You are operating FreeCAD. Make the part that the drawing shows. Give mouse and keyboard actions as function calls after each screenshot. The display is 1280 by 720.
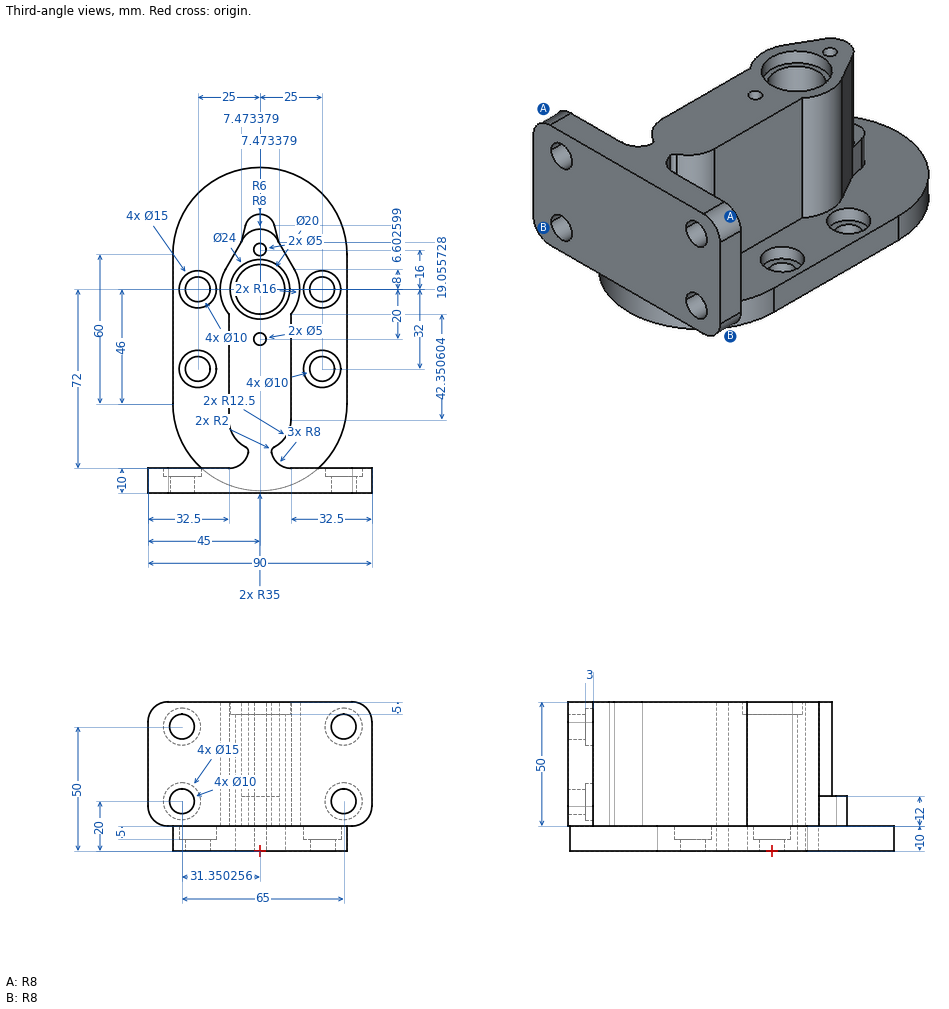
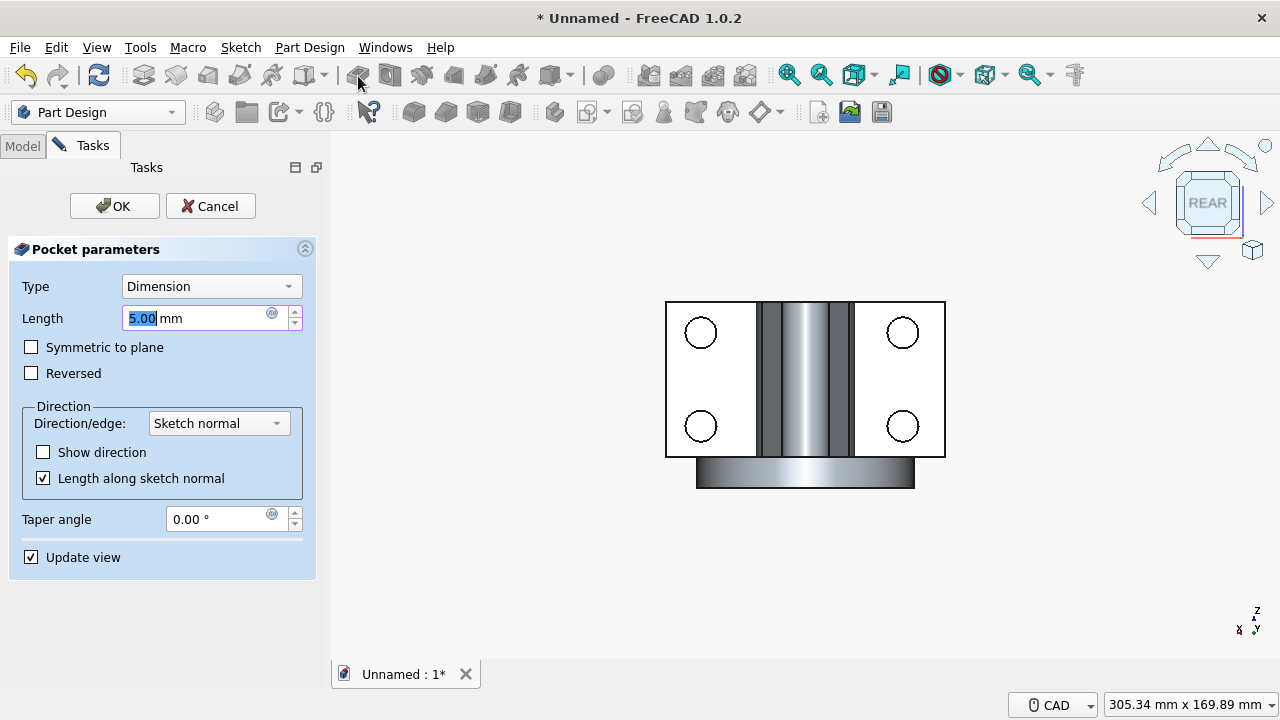
text(20)
key(Tab)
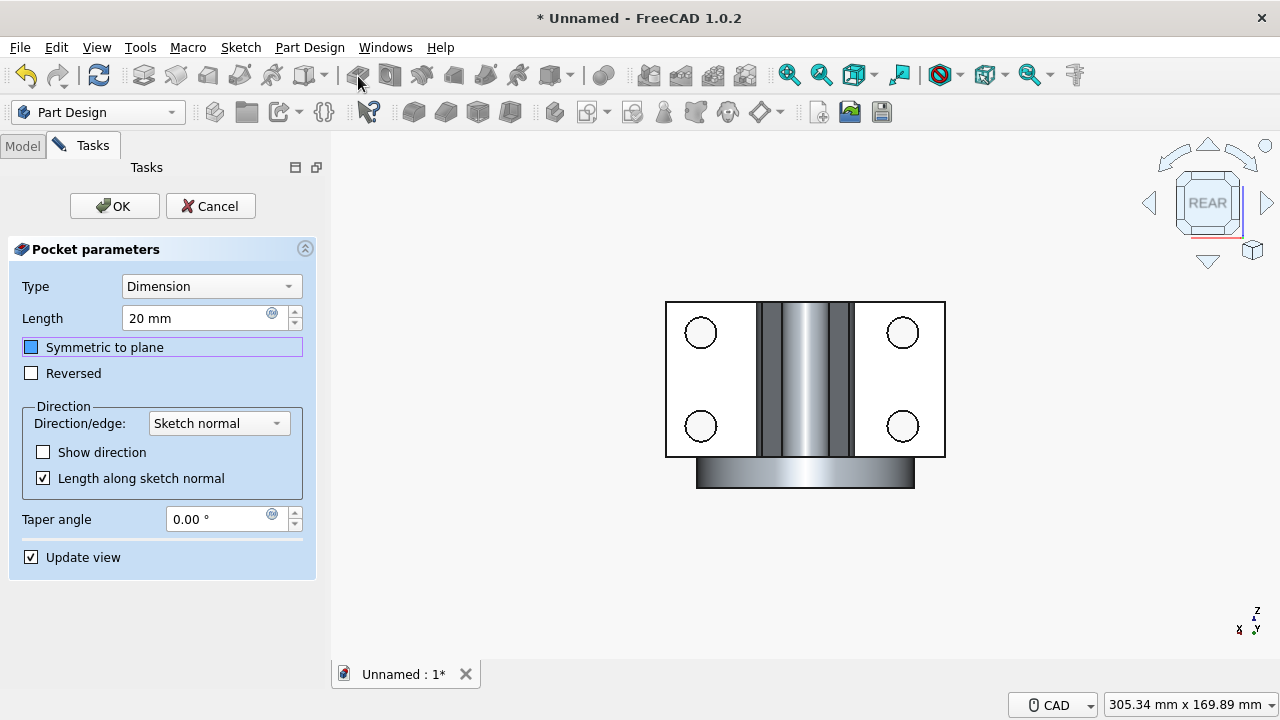
click(115, 206)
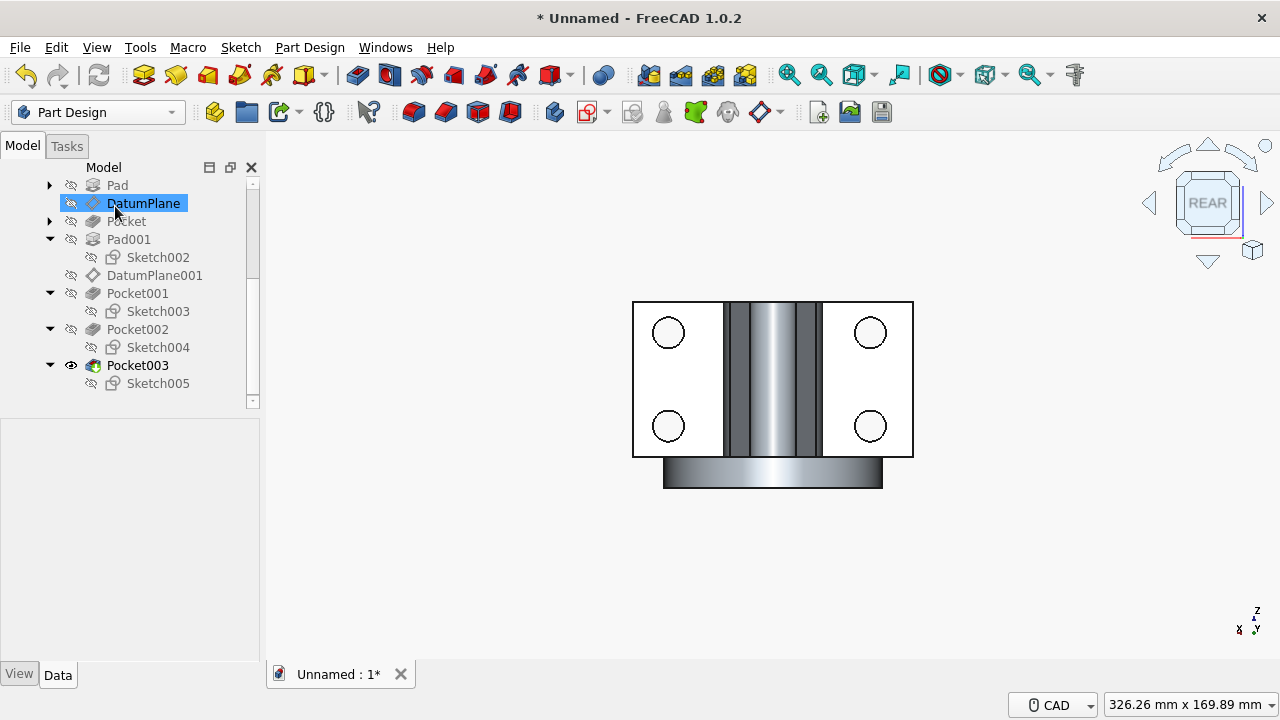
click(790, 76)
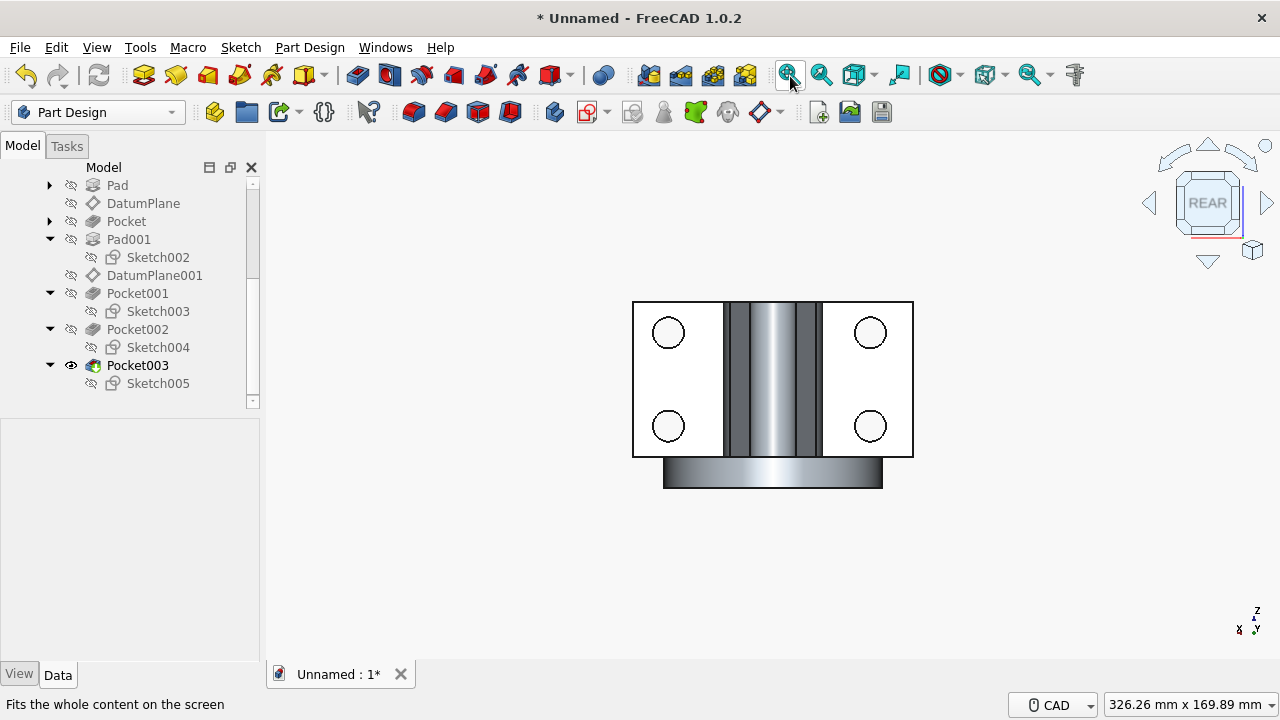
click(848, 378)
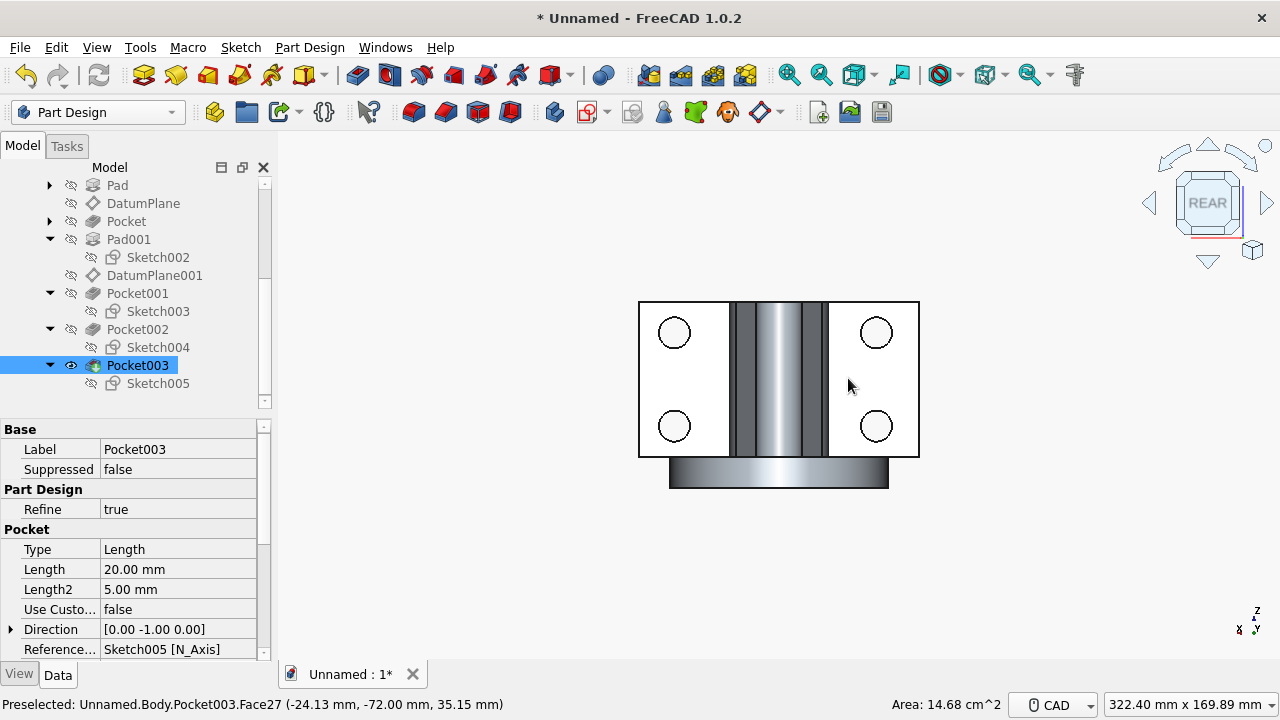
click(588, 112)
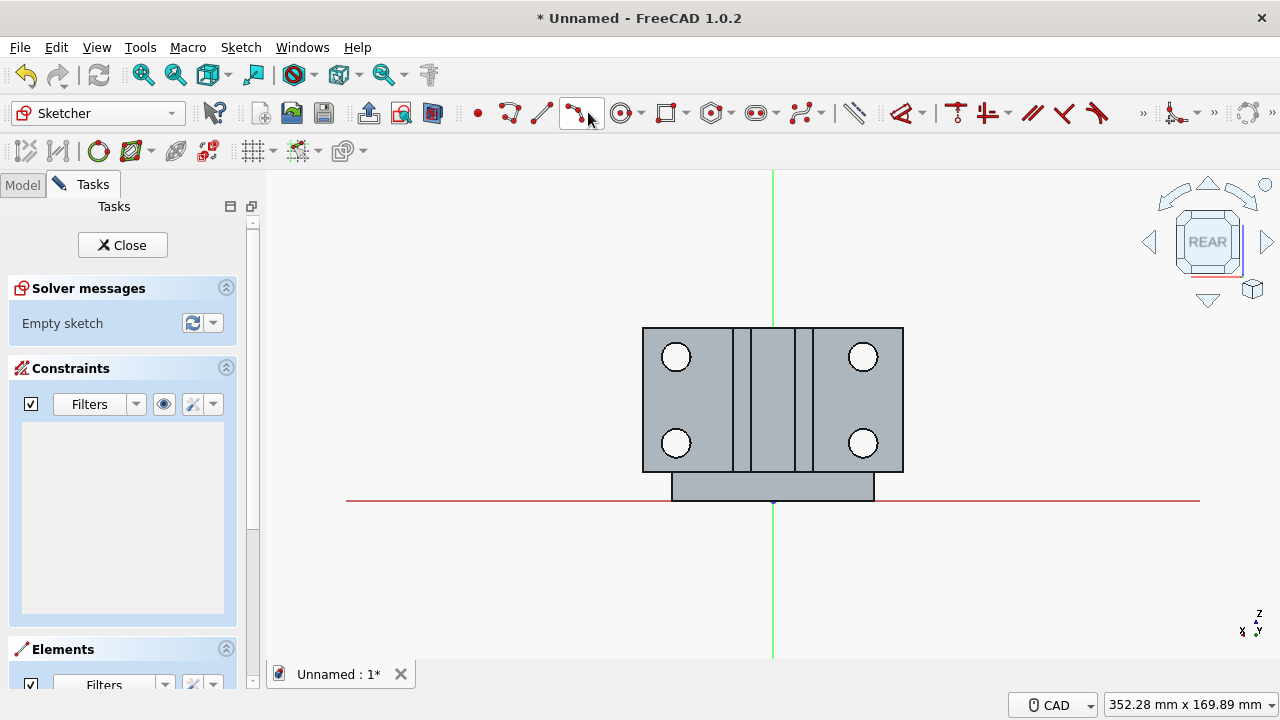
scroll(849, 422, up, 3)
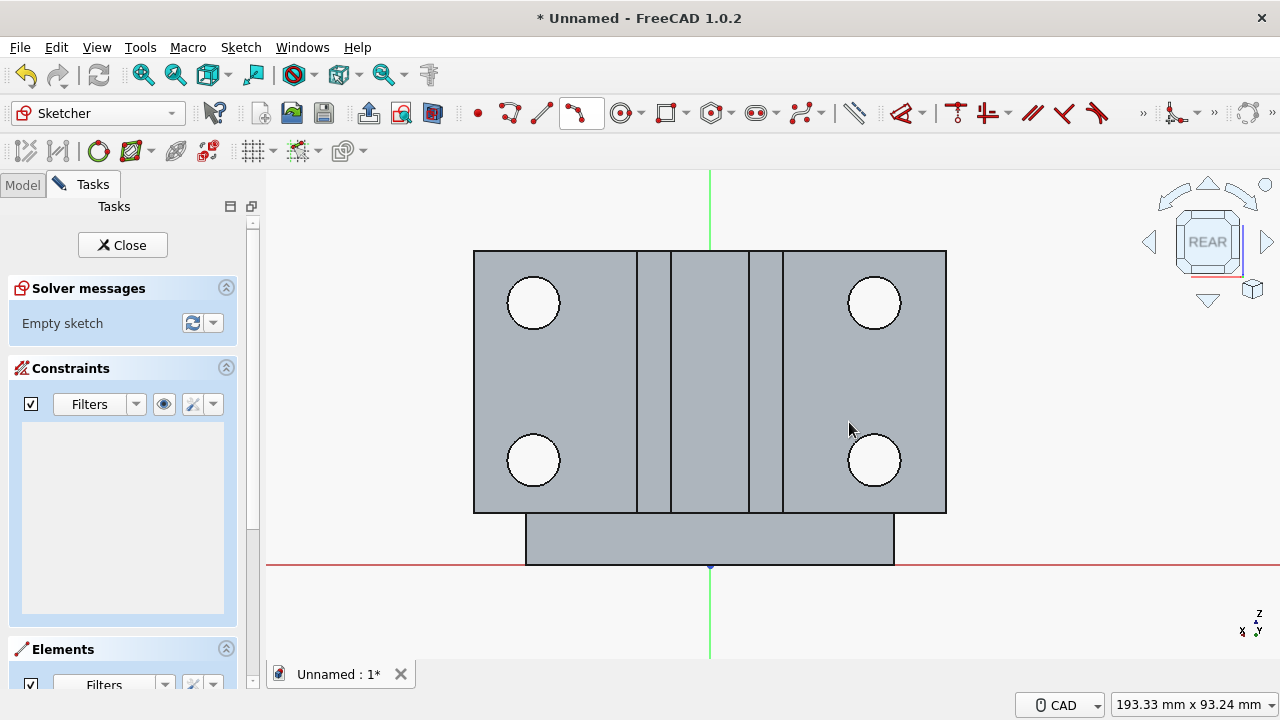
click(622, 114)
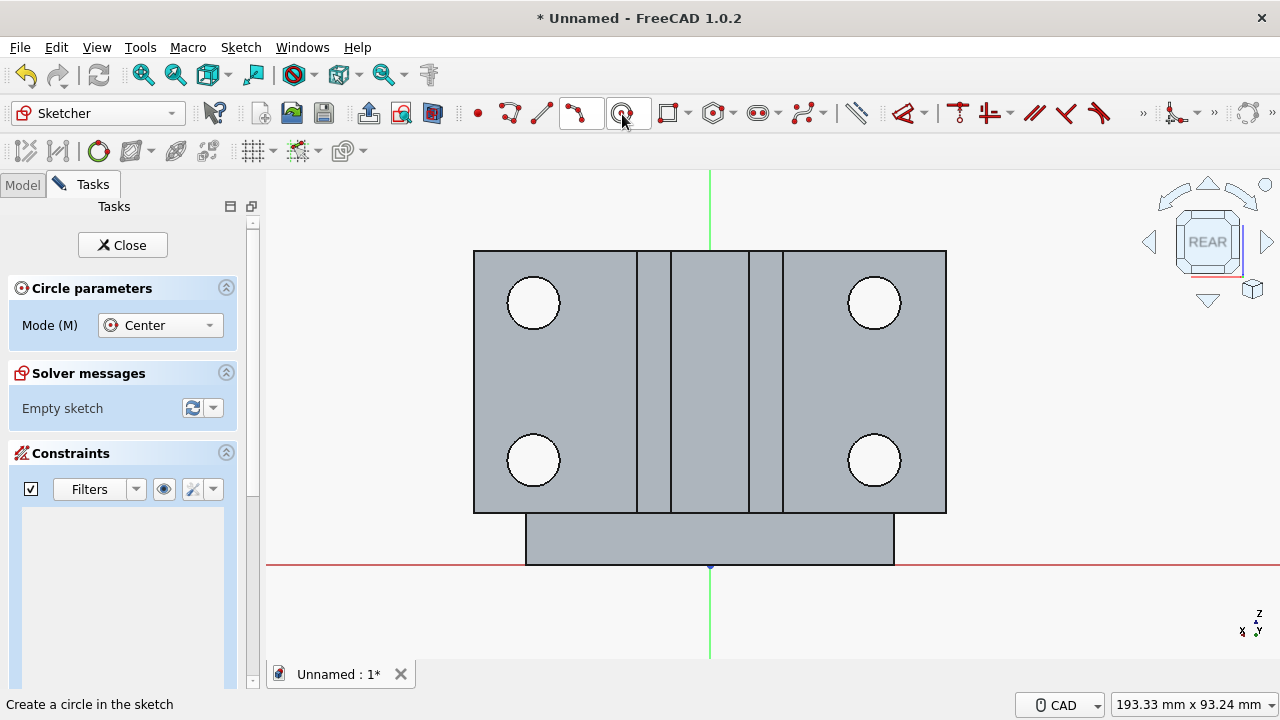
click(874, 460)
click(902, 433)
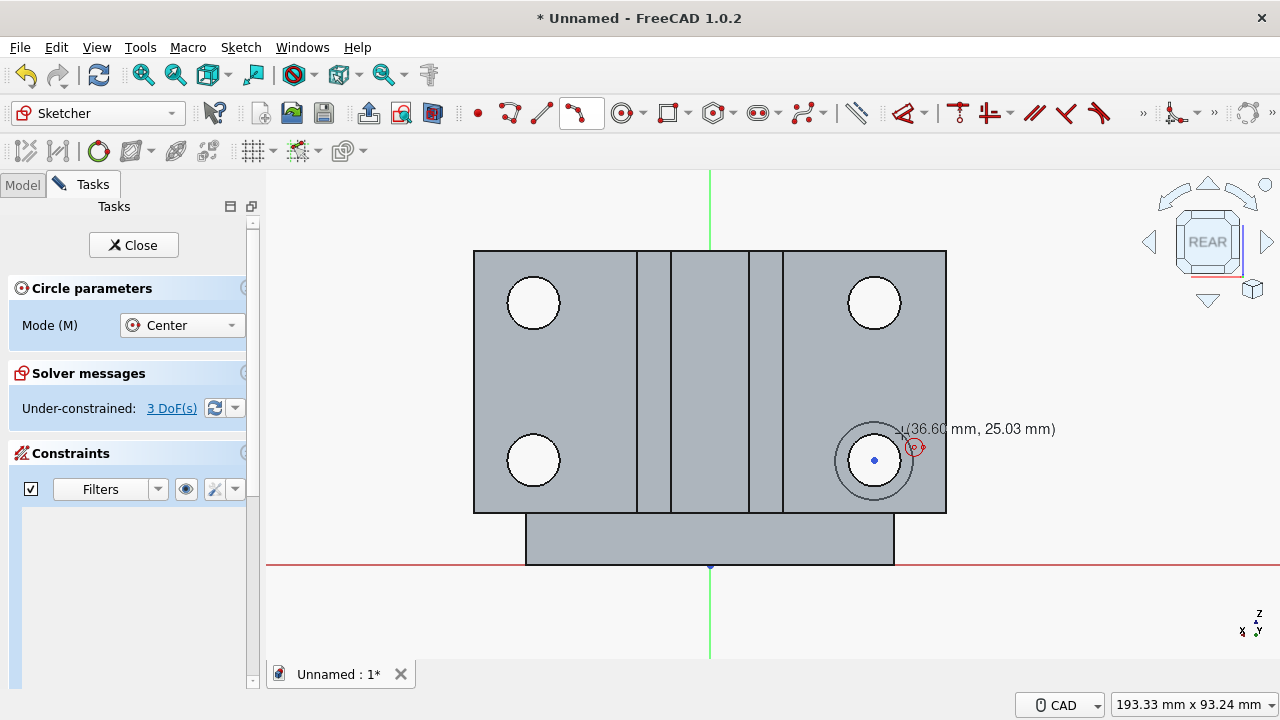
click(874, 303)
click(902, 275)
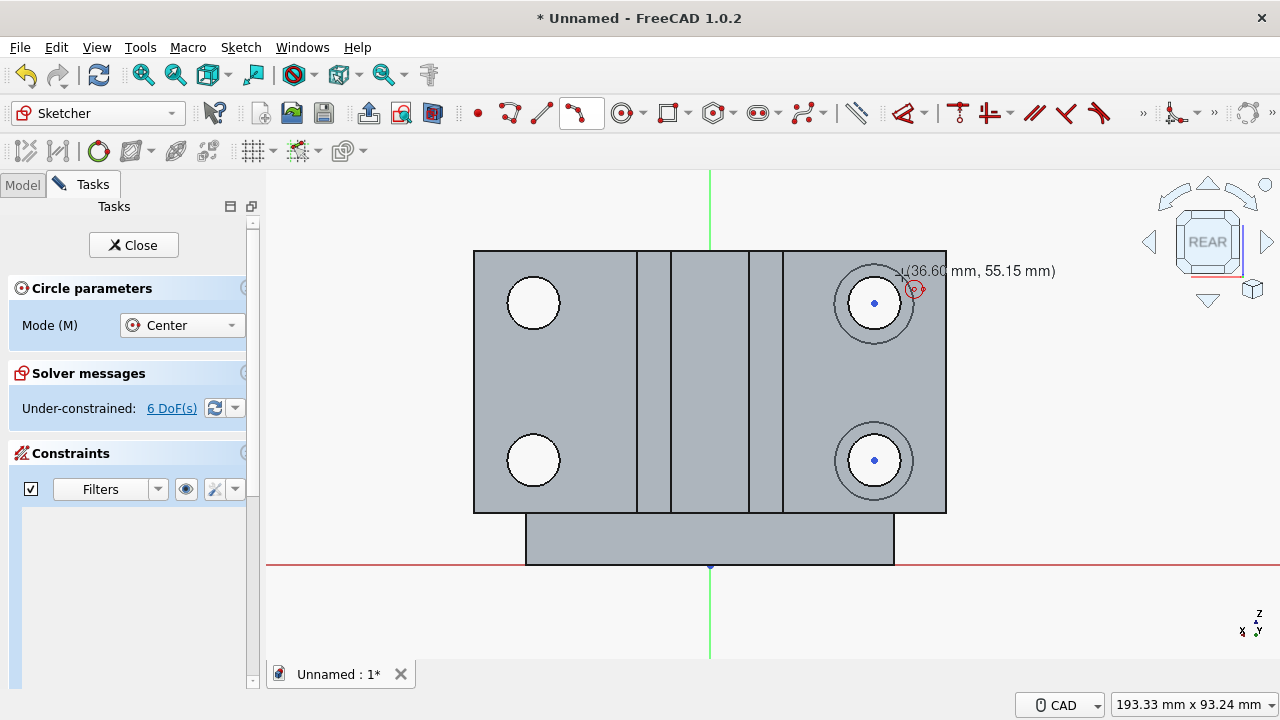
click(534, 460)
click(561, 433)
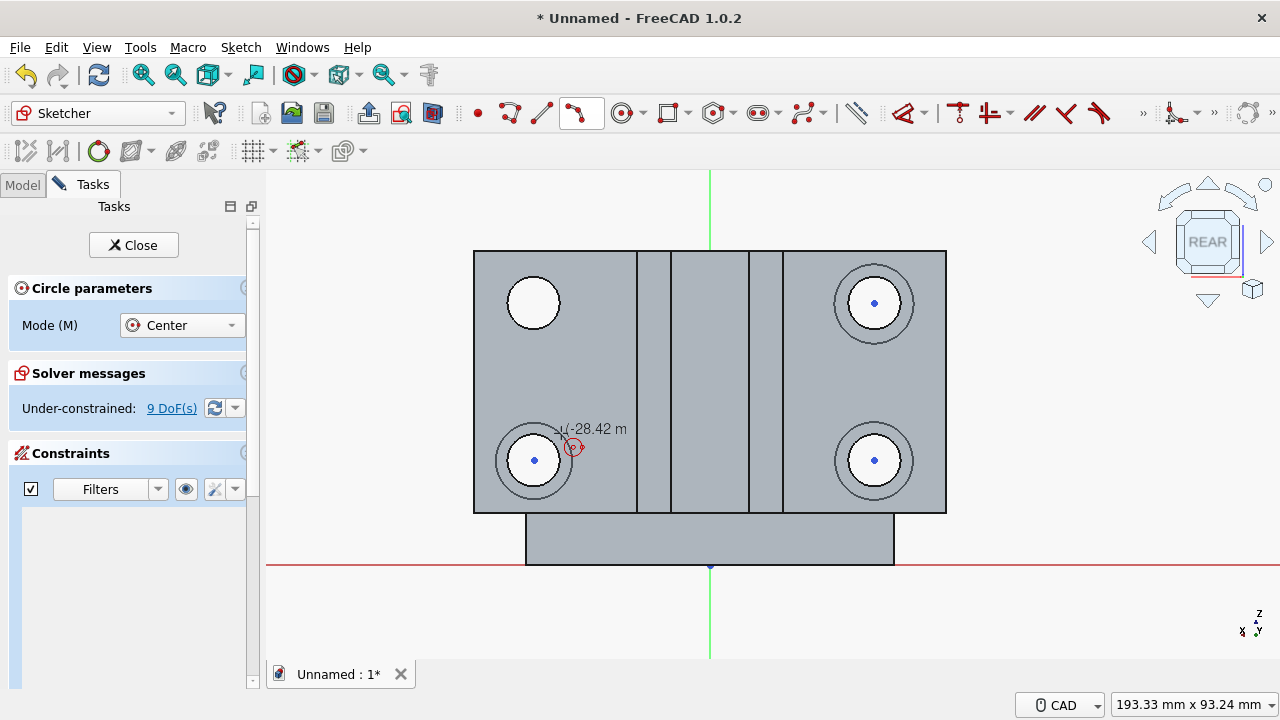
click(534, 303)
click(561, 275)
key(Escape)